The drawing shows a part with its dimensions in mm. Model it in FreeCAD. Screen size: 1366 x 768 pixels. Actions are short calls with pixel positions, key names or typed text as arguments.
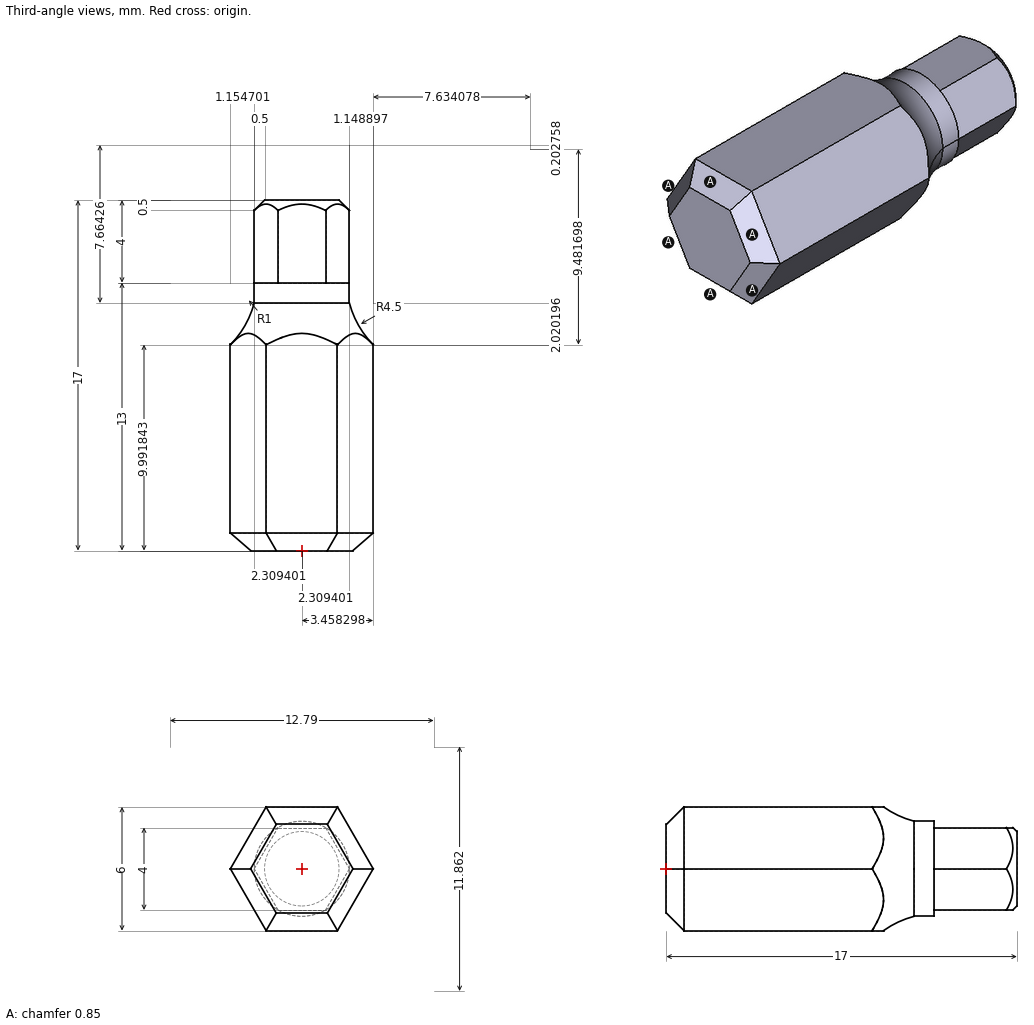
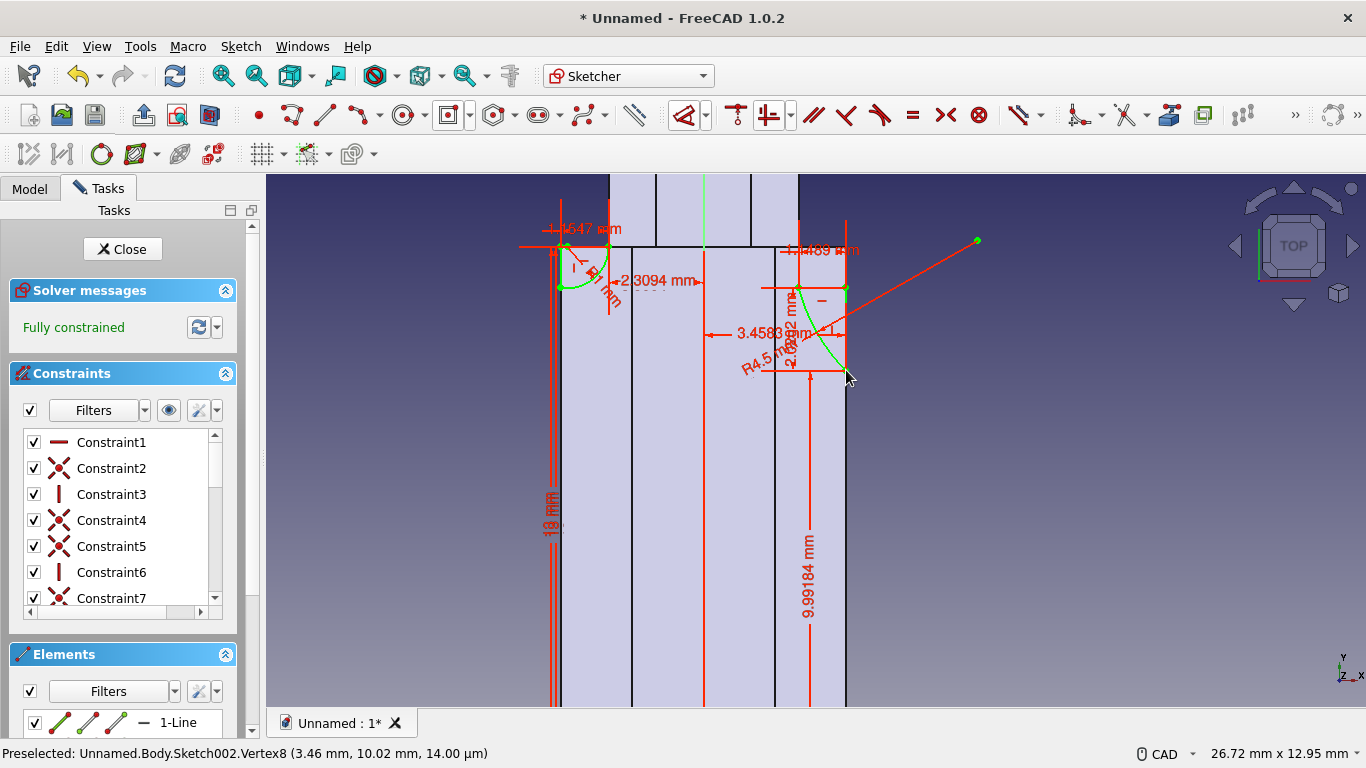
click(123, 249)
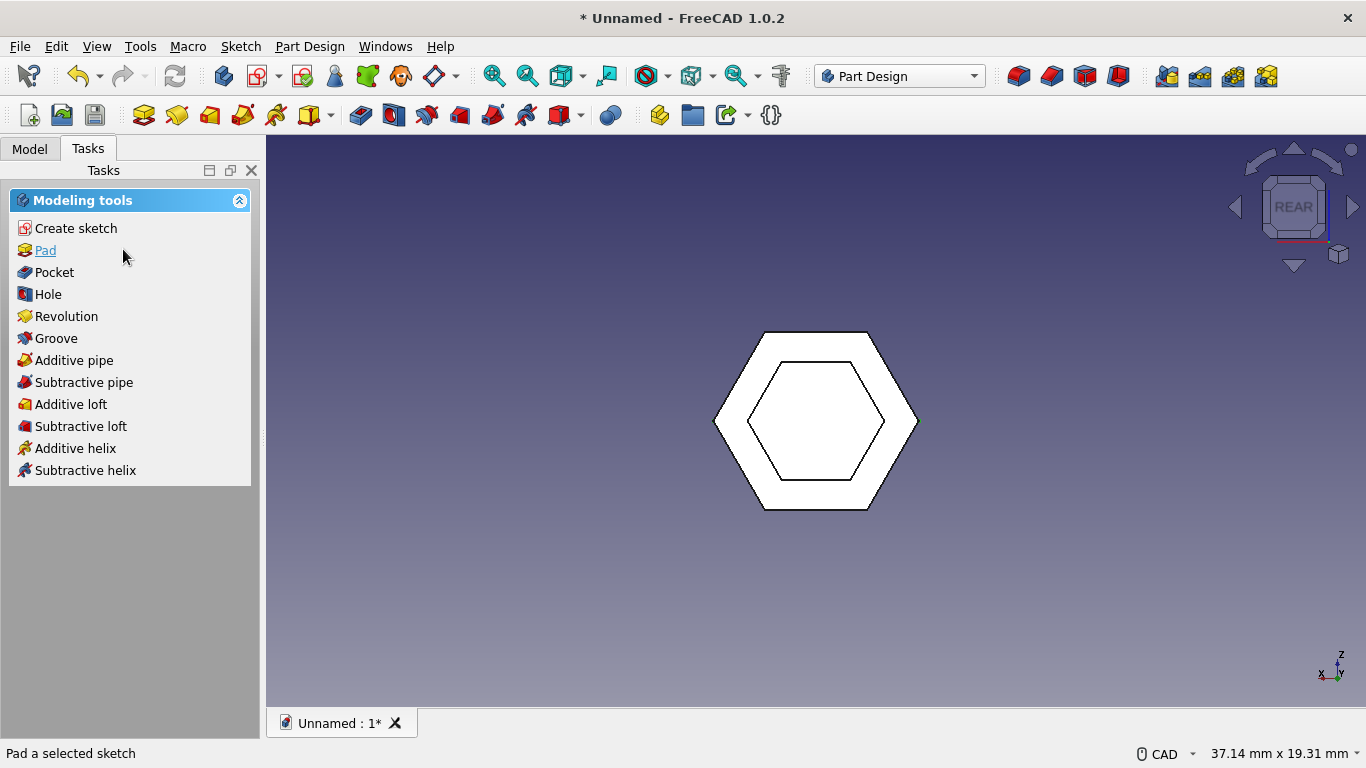
click(427, 116)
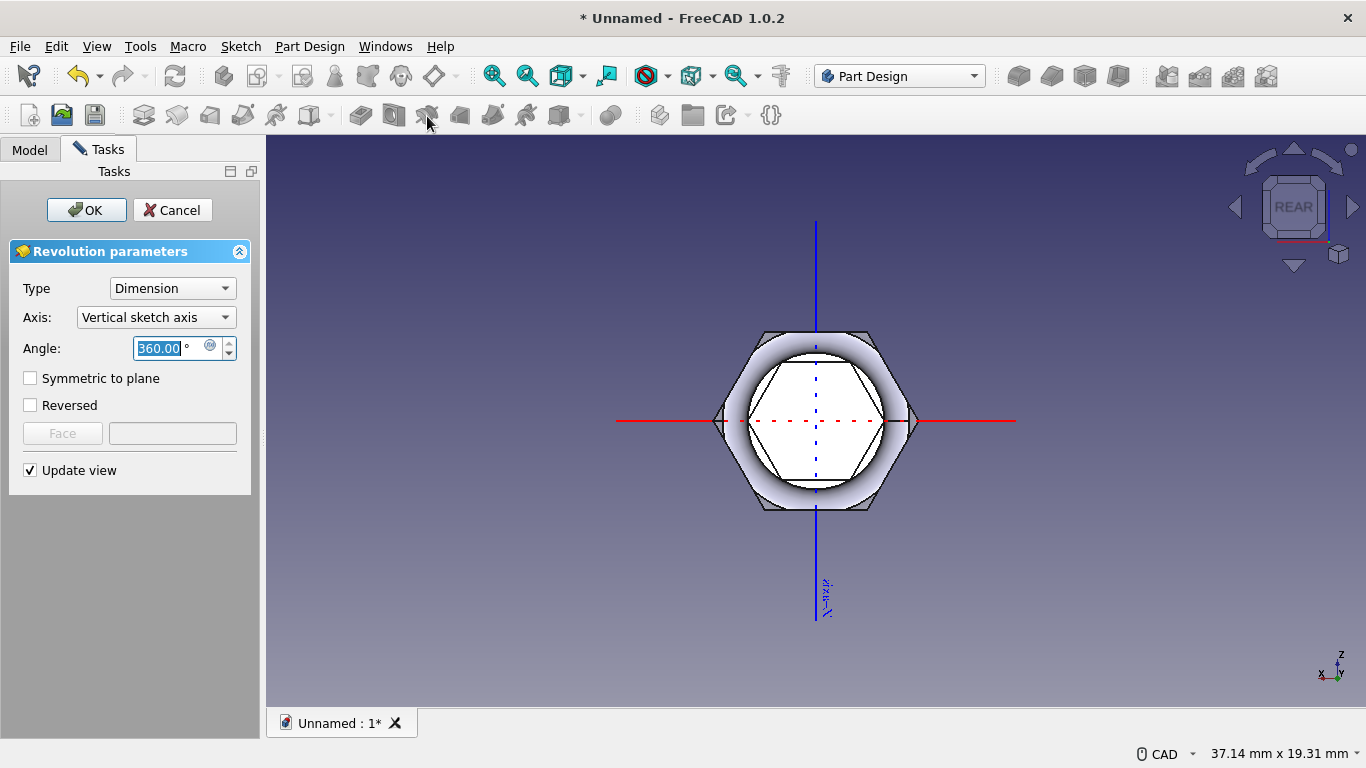
click(87, 210)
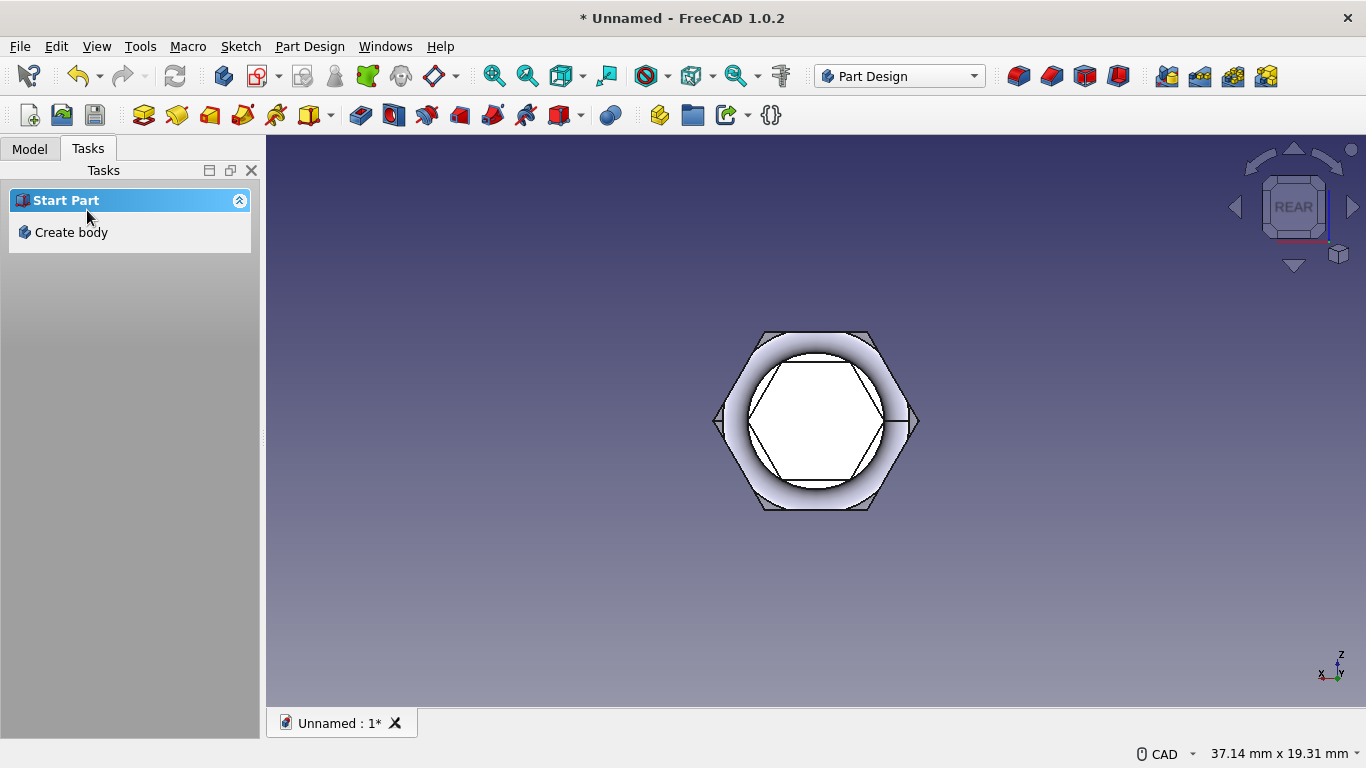
click(495, 76)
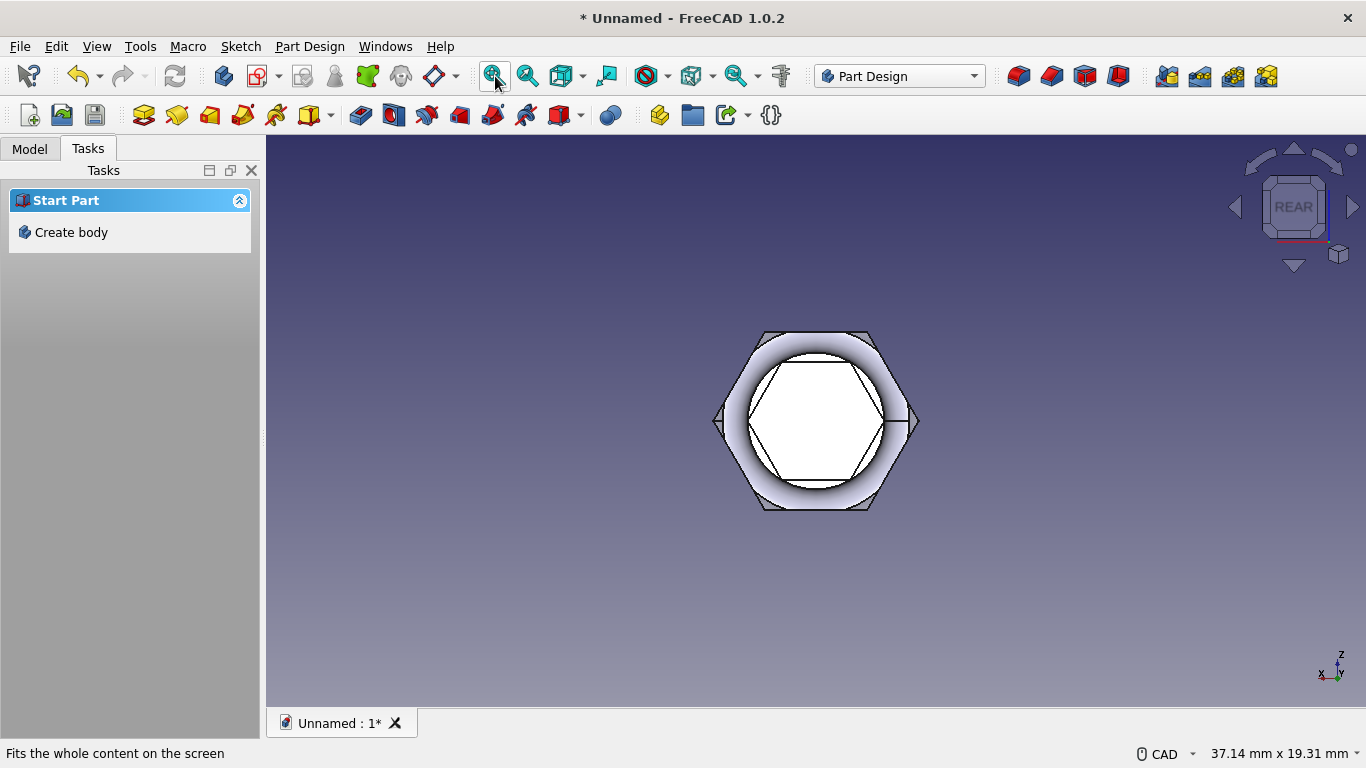
click(256, 76)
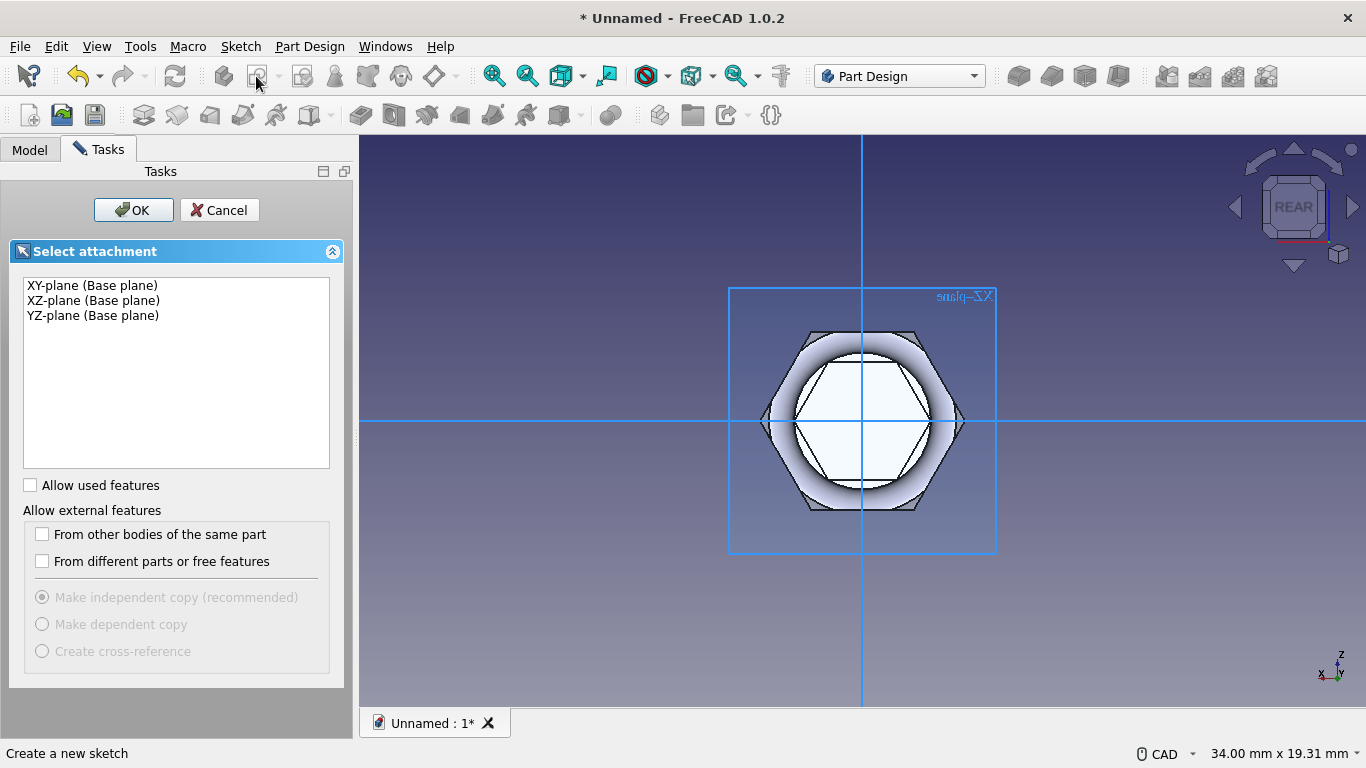
click(84, 286)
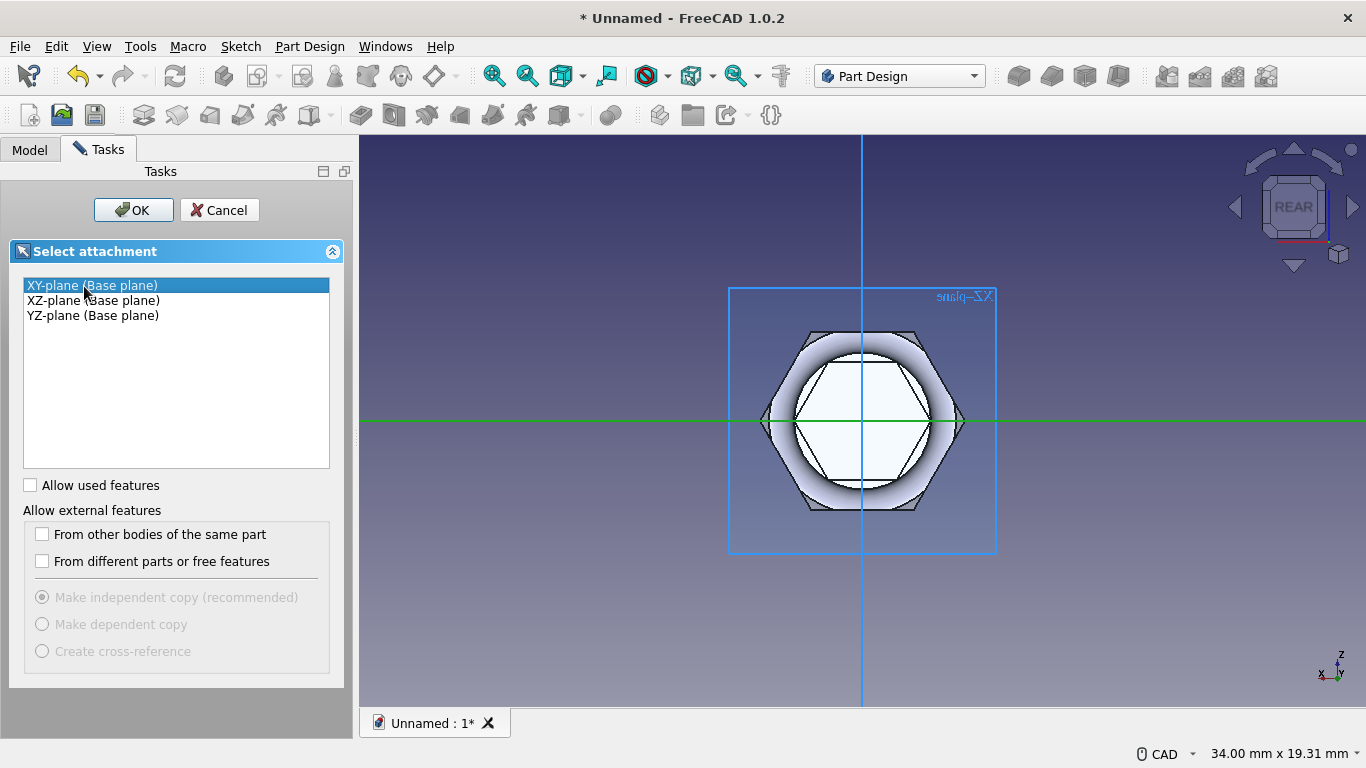
click(134, 210)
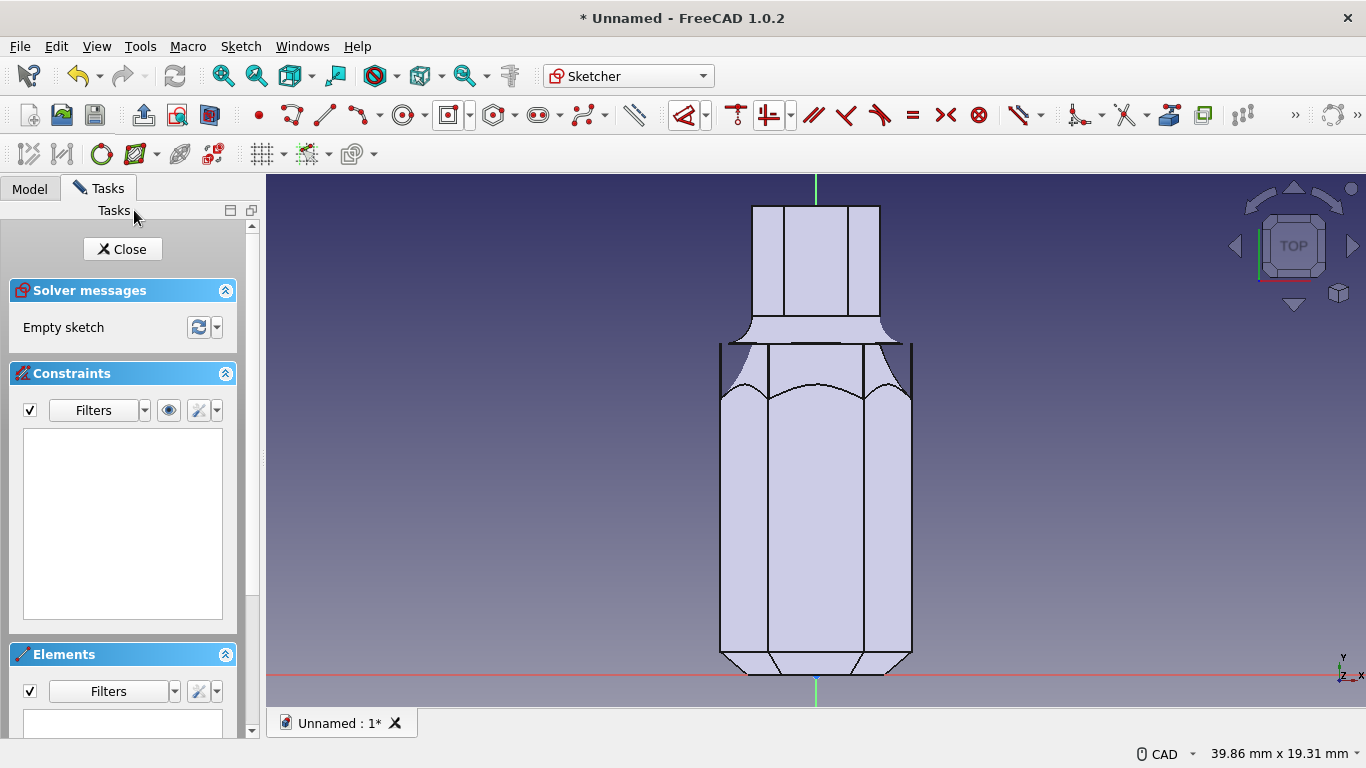
click(210, 116)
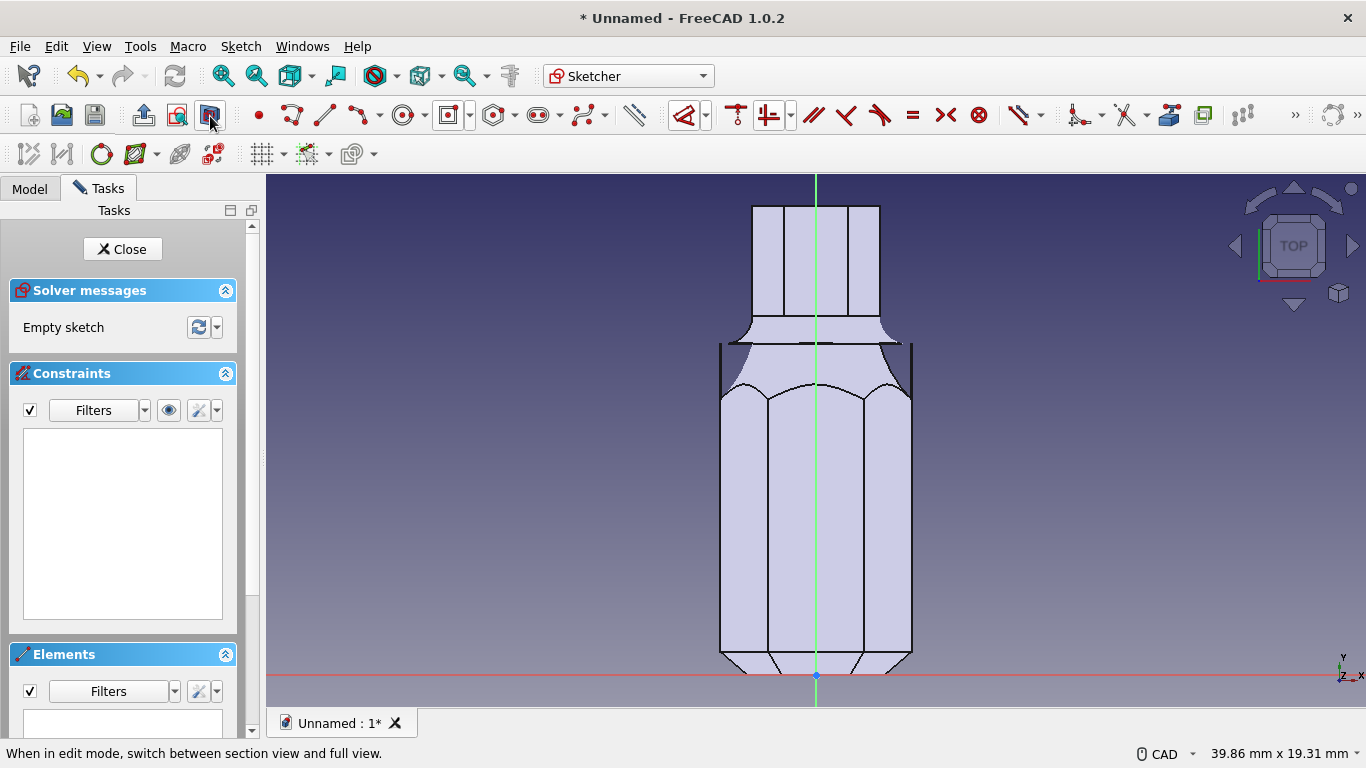
scroll(297, 516, down, 2)